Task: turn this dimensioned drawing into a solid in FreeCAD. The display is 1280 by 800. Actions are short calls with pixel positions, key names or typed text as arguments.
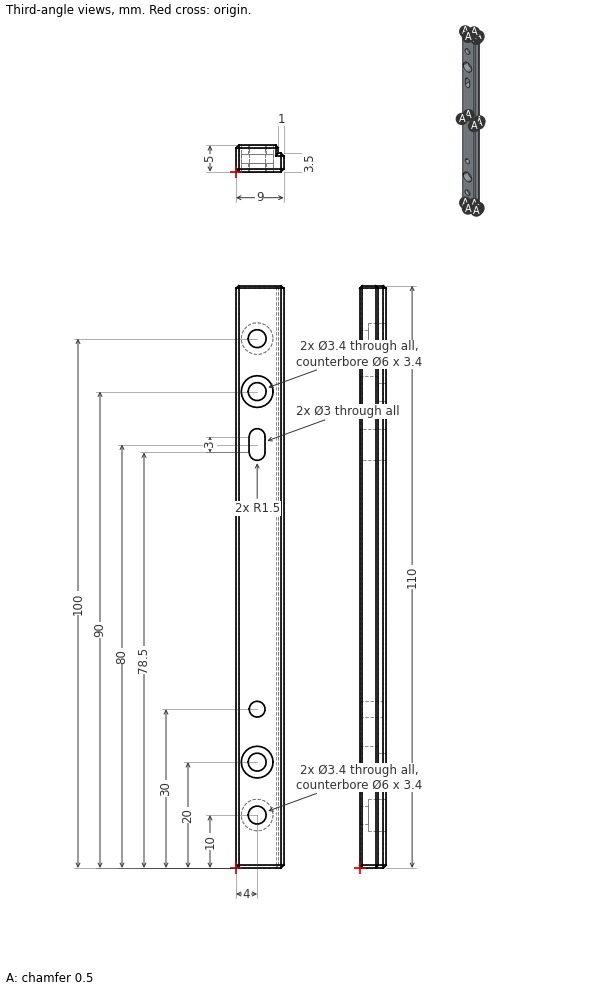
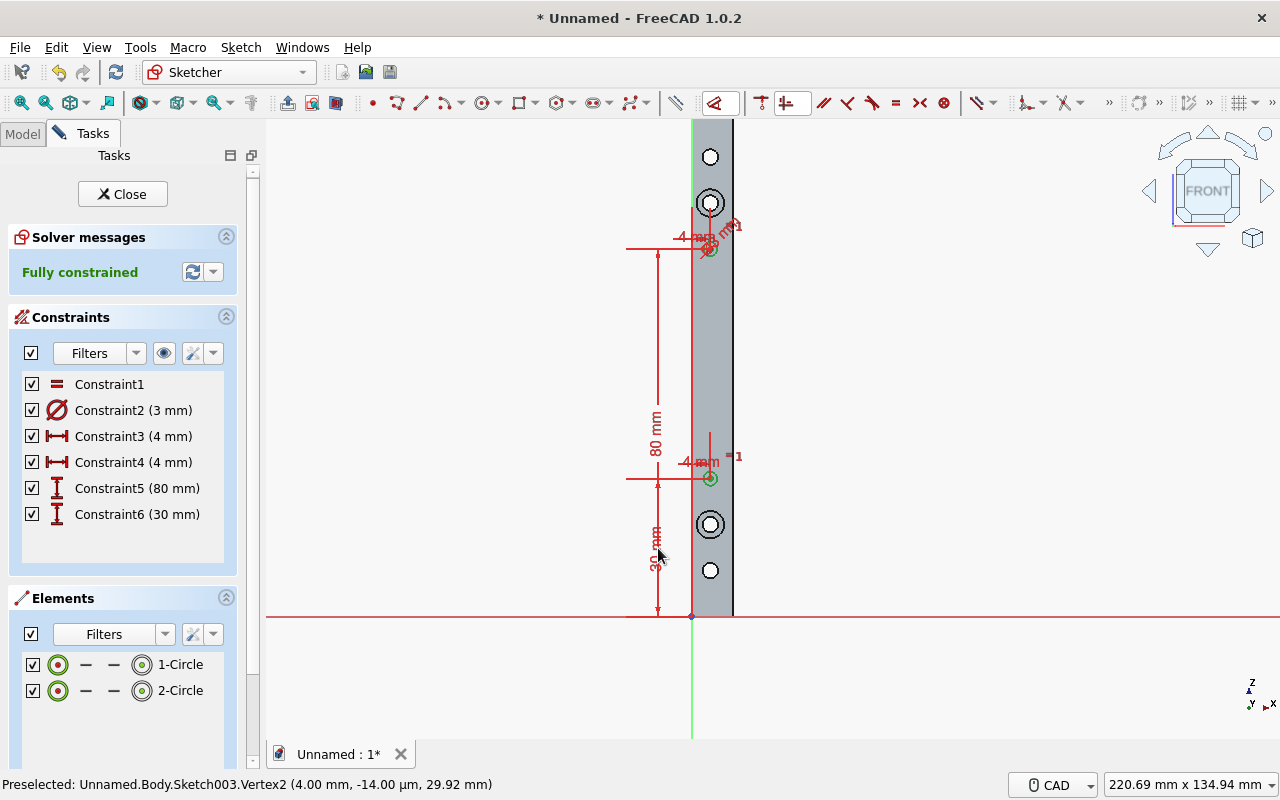
click(123, 194)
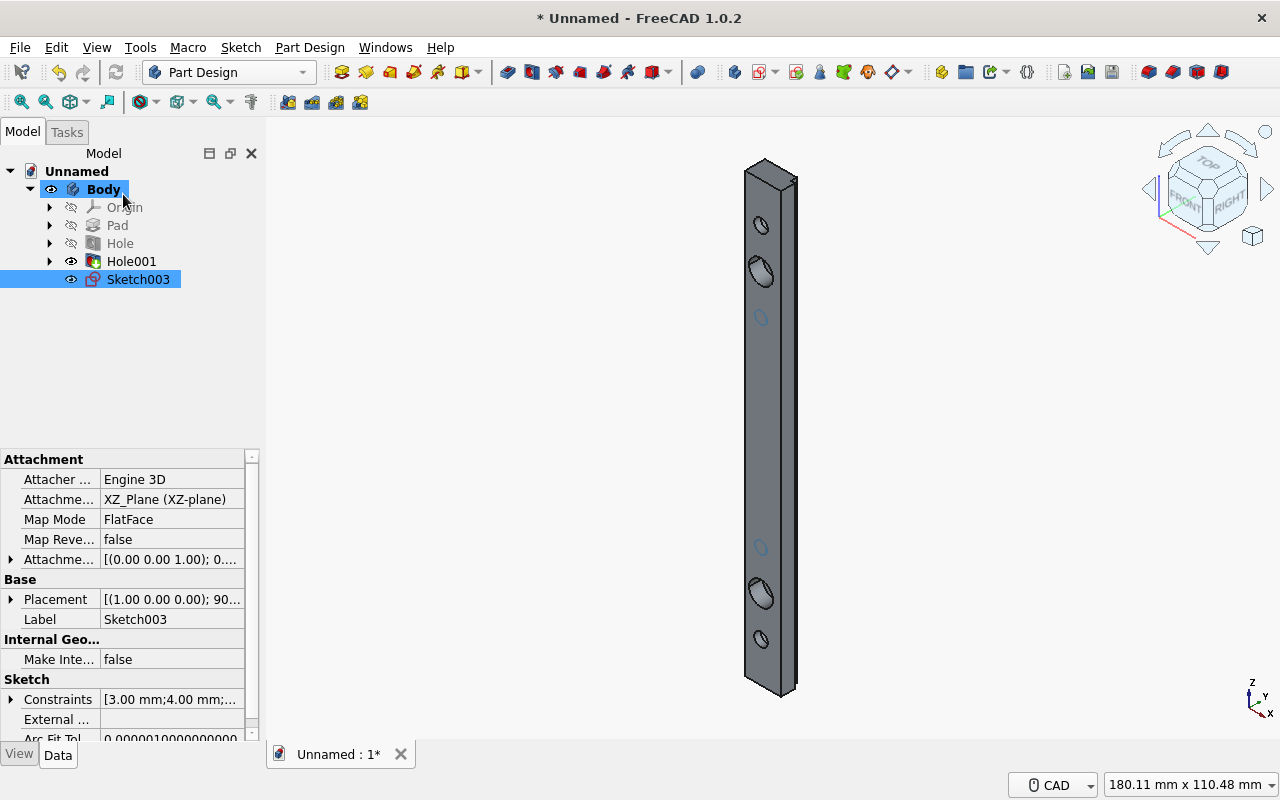
click(532, 72)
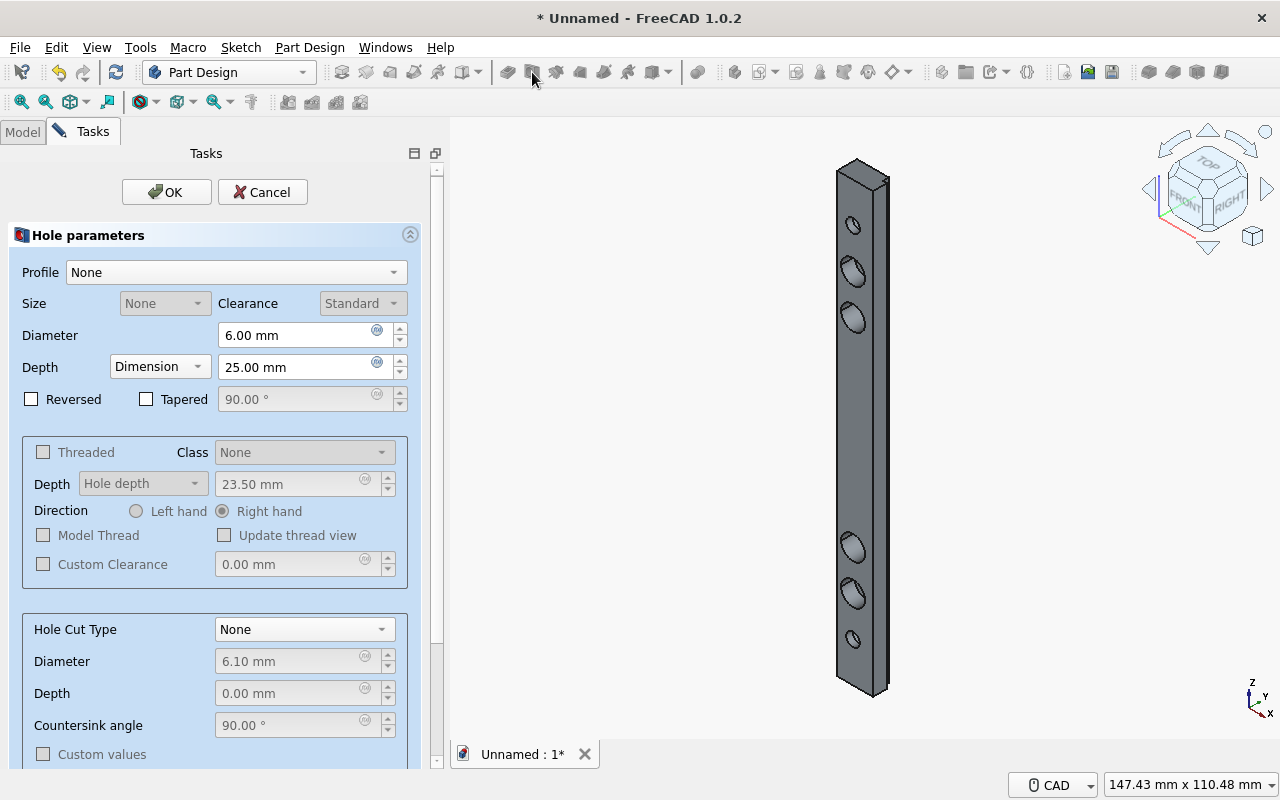
triple_click(305, 335)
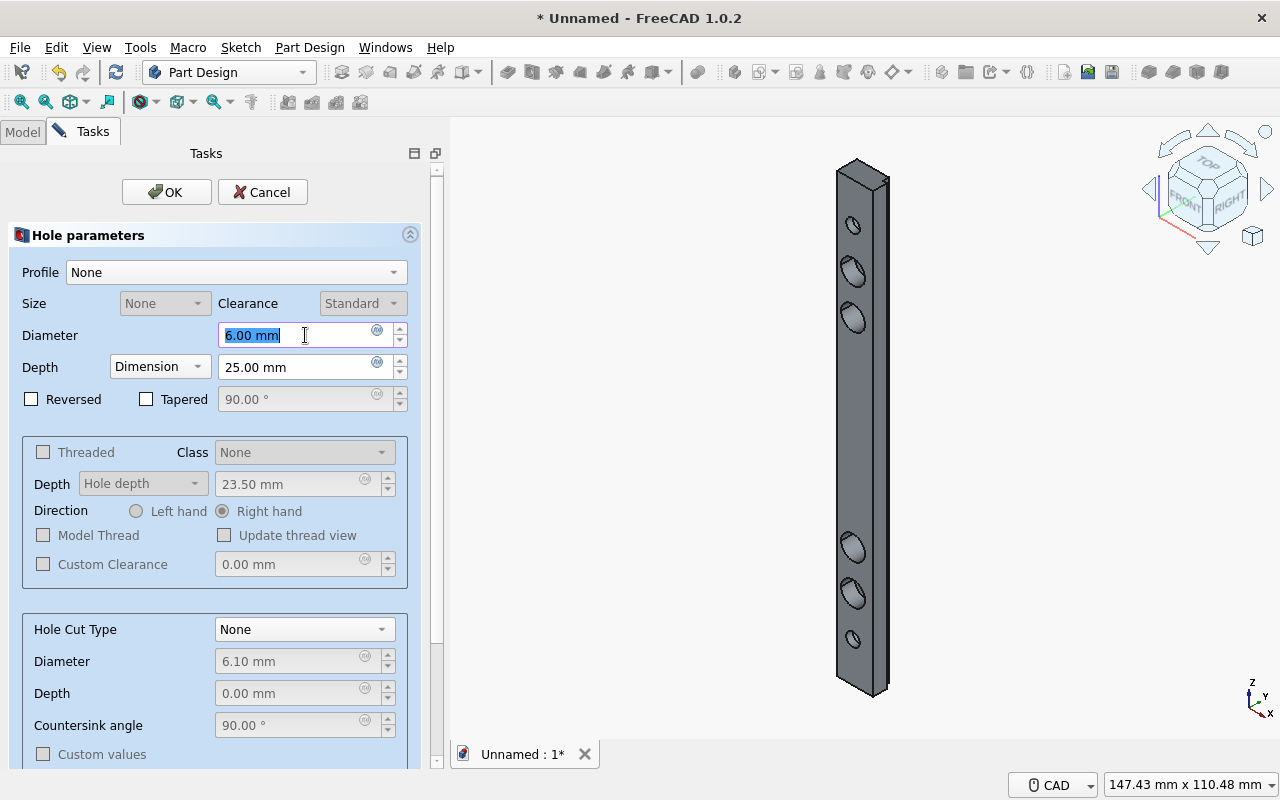
text(3)
key(Tab)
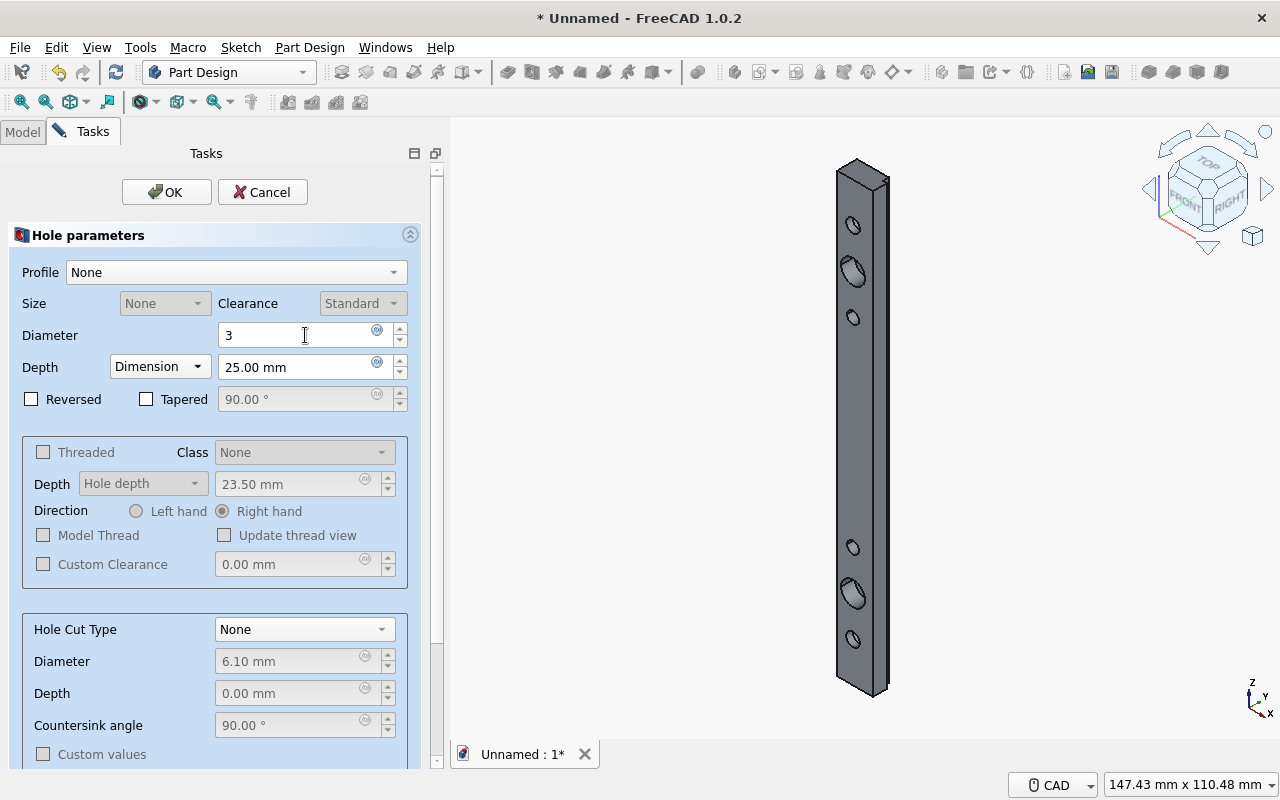
click(161, 366)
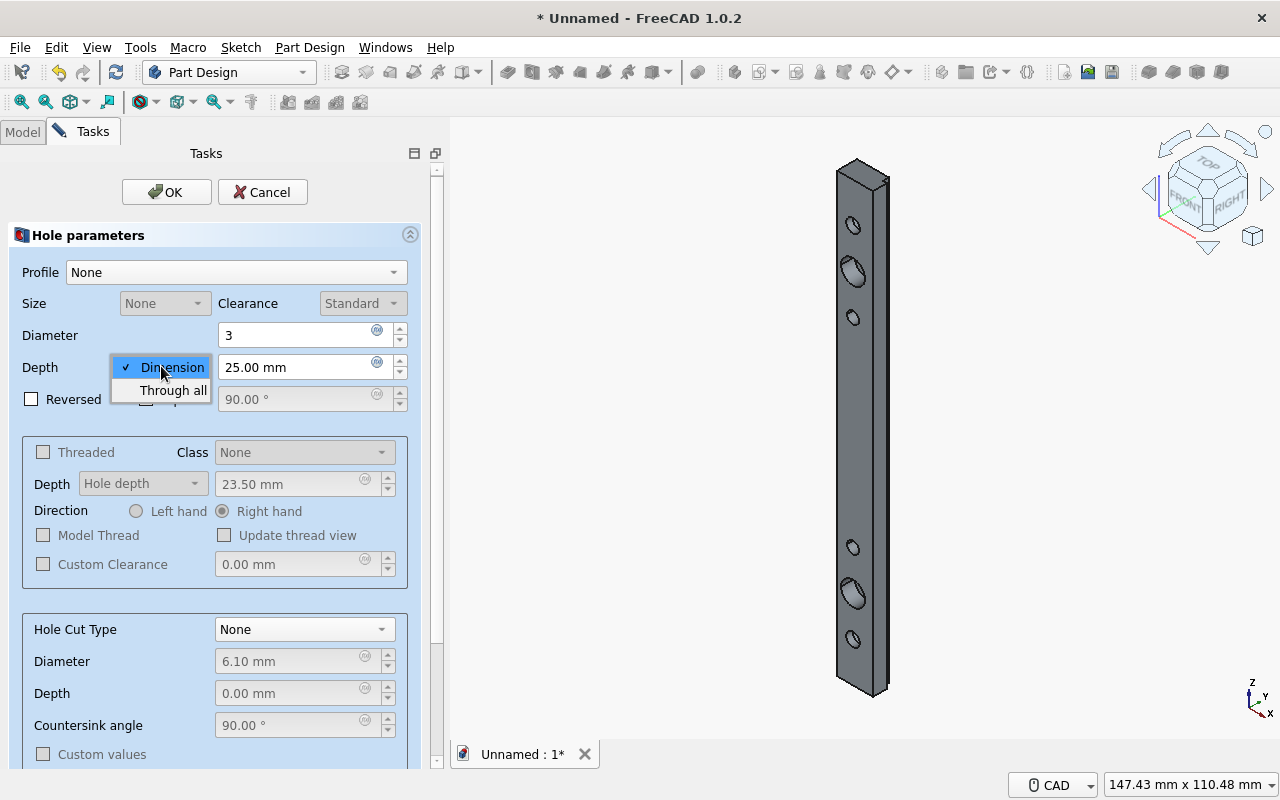
click(160, 390)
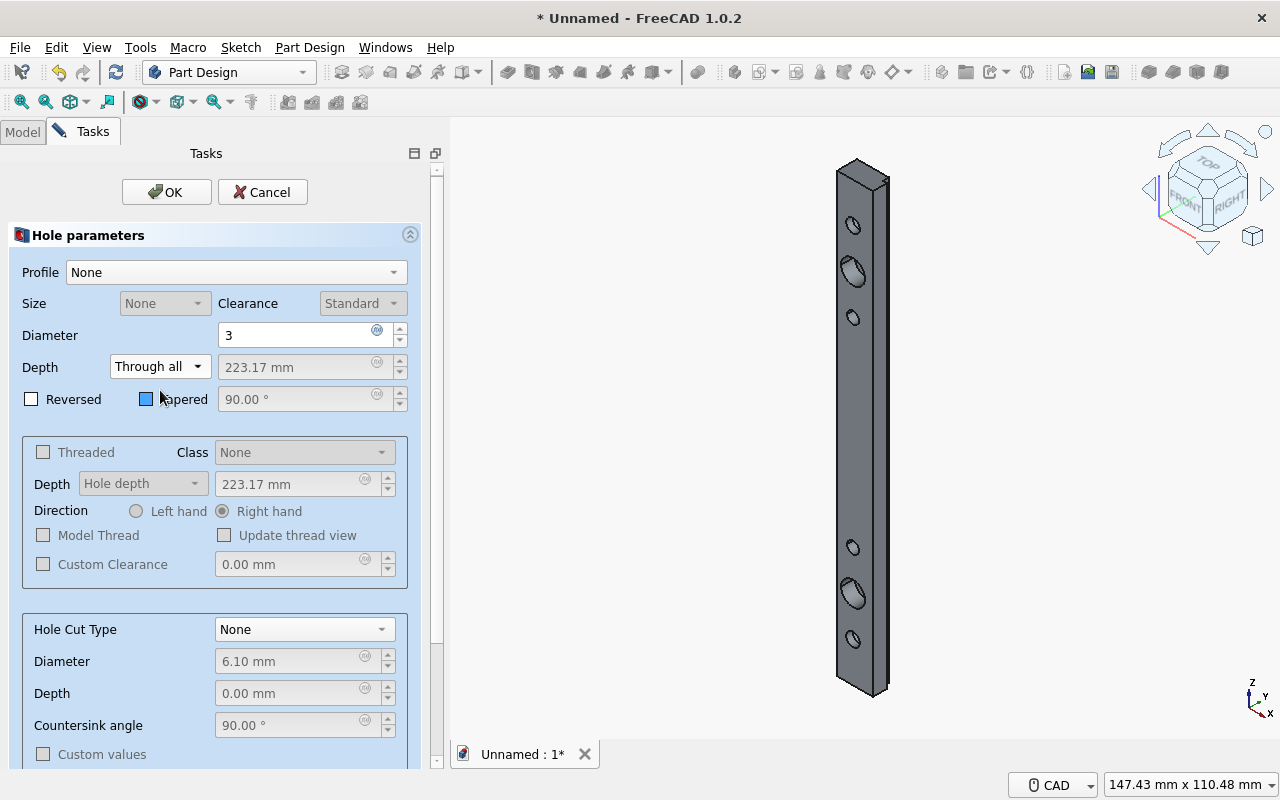
click(167, 192)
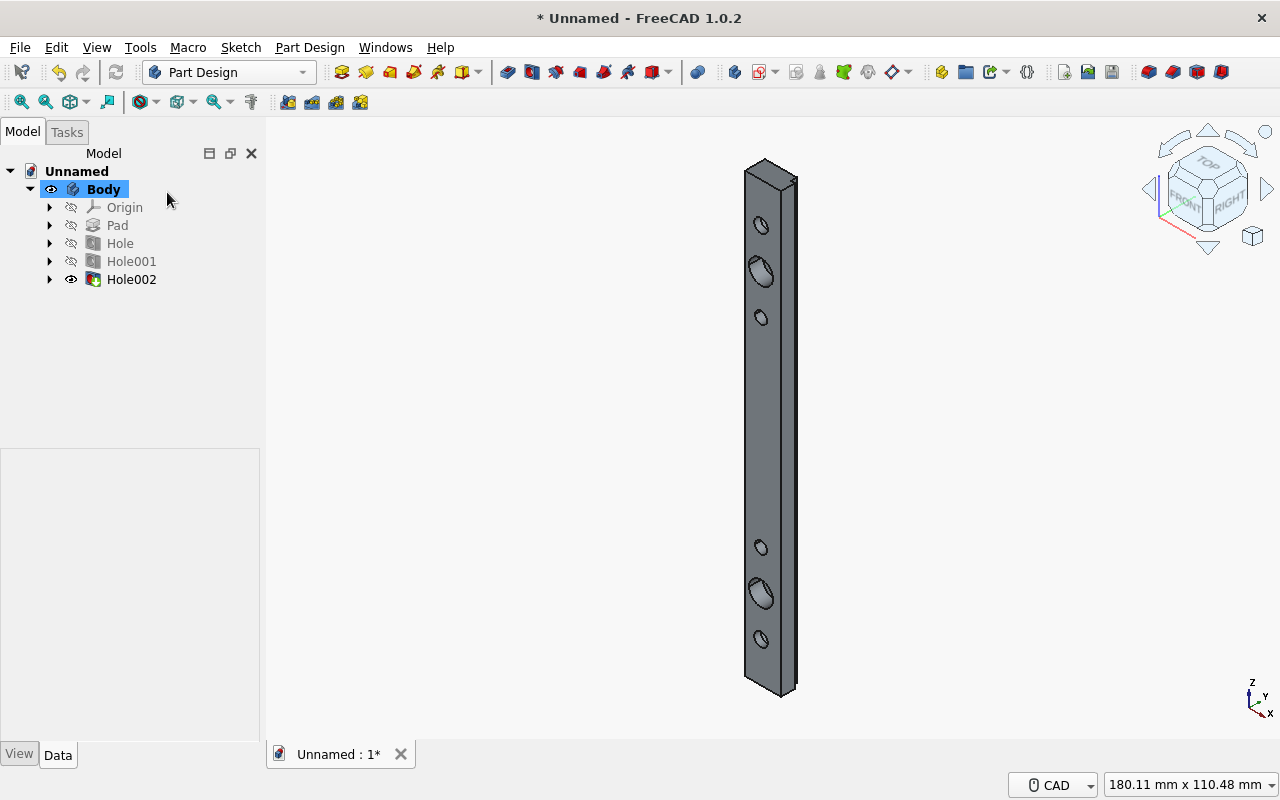
click(760, 72)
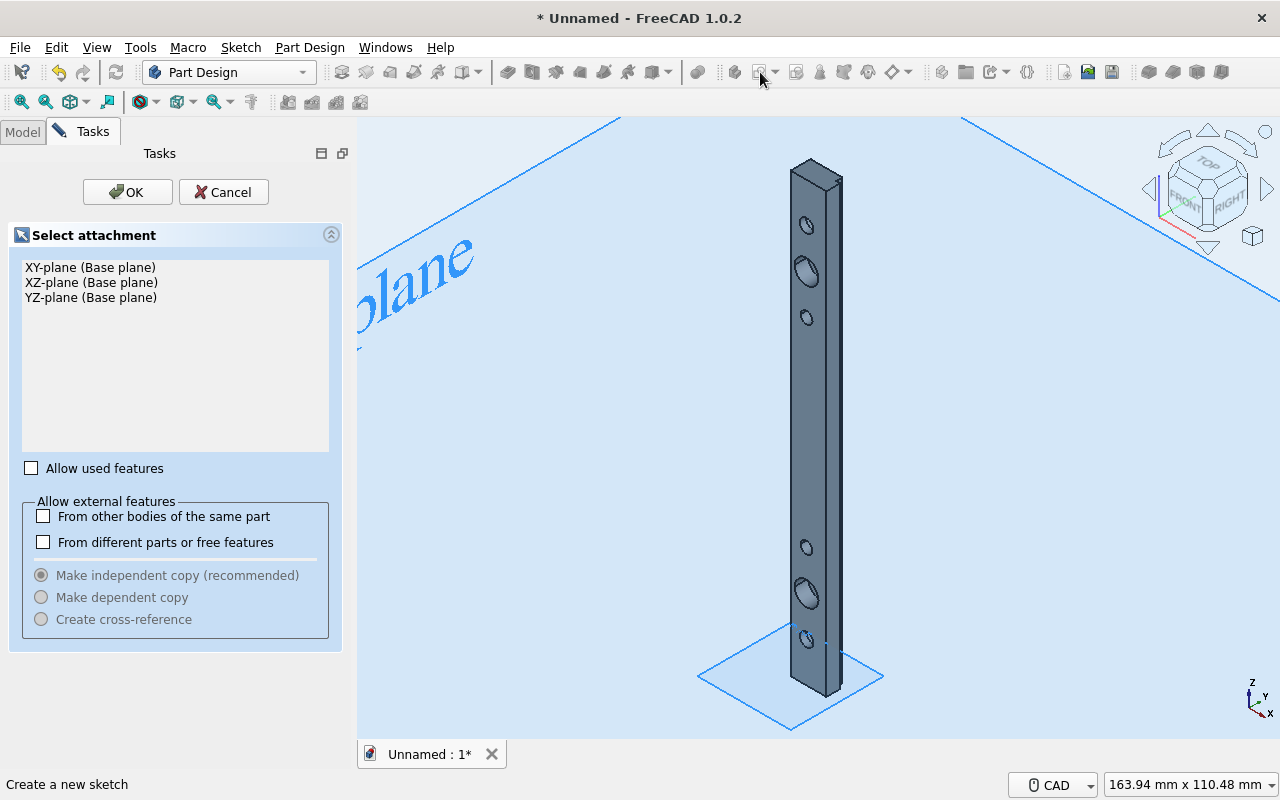
click(82, 282)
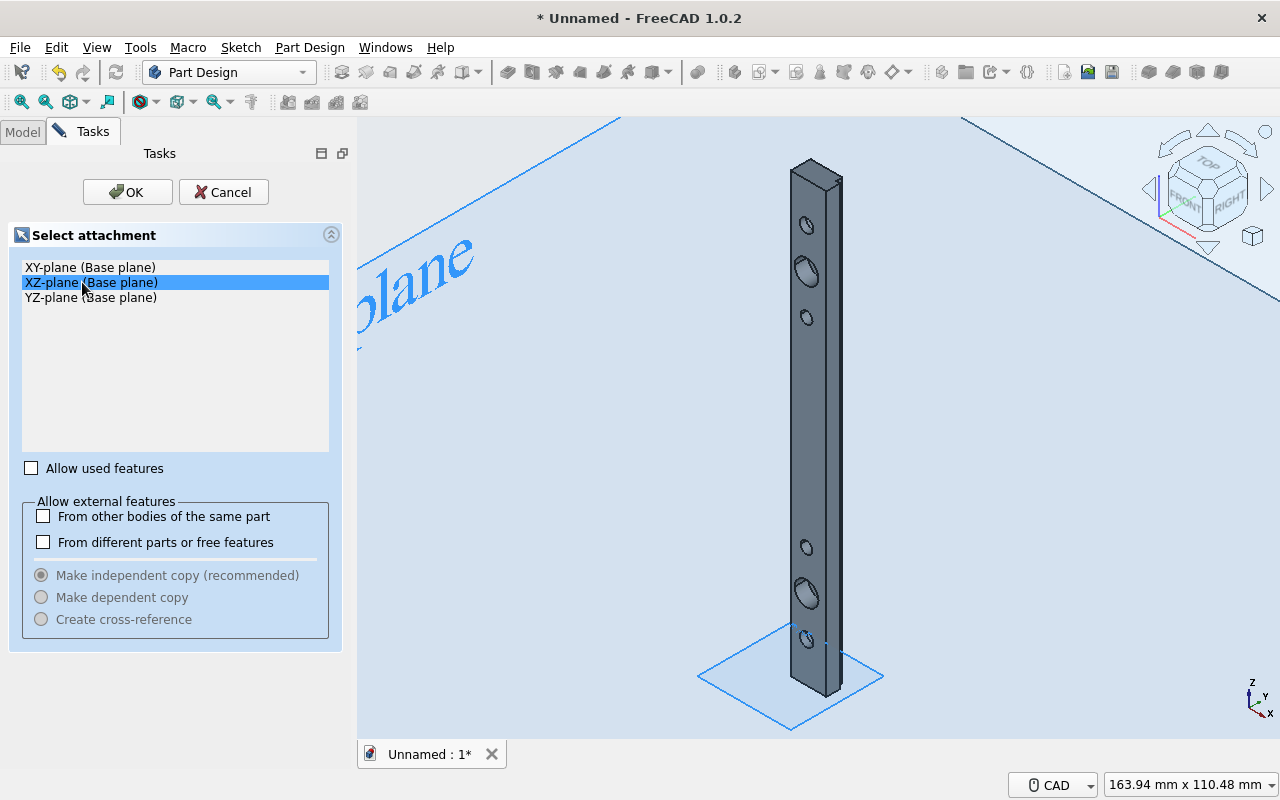
click(128, 192)